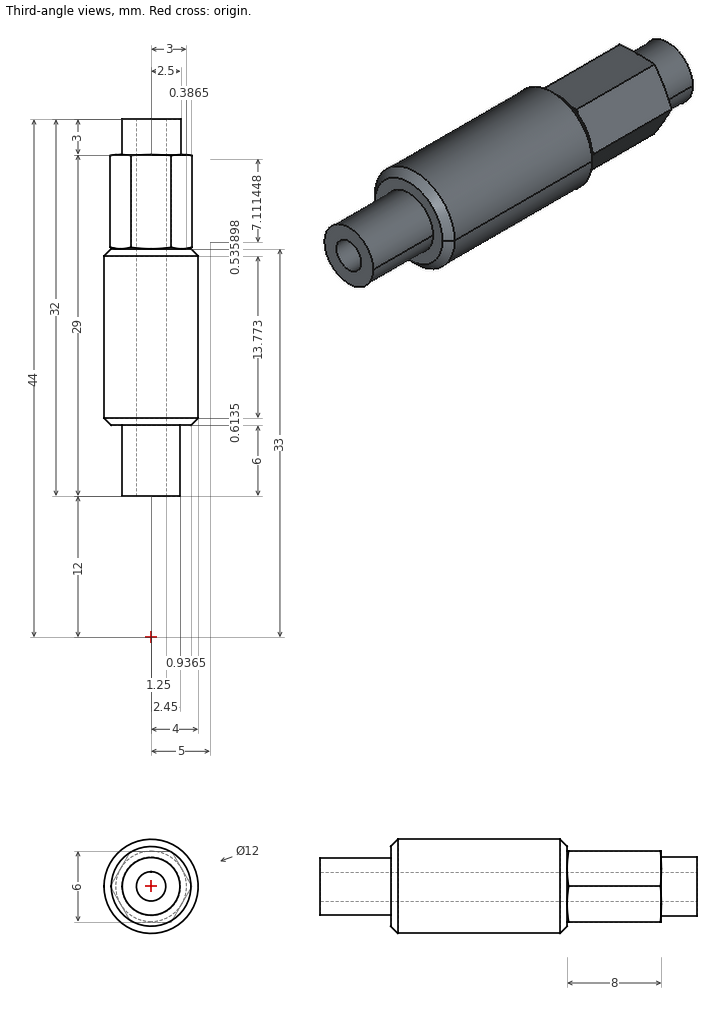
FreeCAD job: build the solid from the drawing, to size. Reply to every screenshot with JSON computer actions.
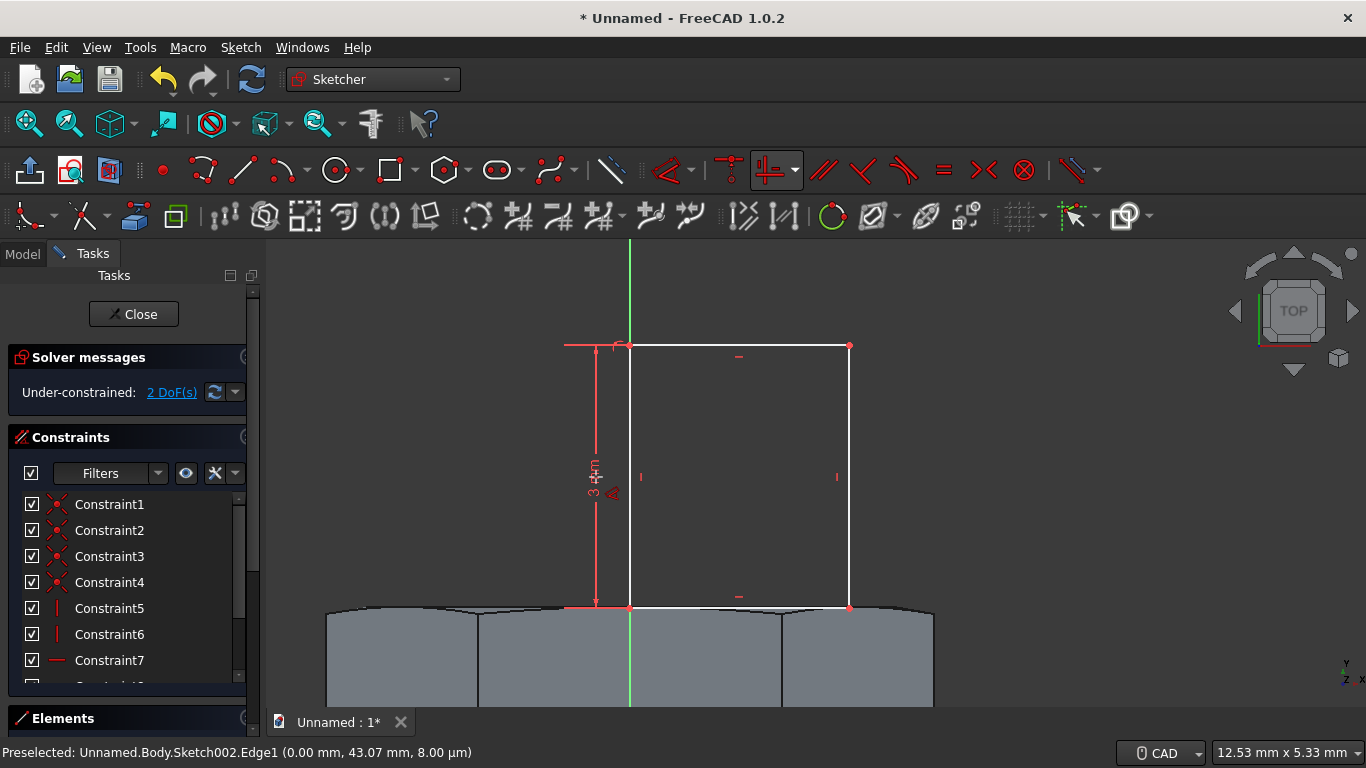
{"action": "left_click", "coordinate": [696, 608]}
{"action": "left_click", "coordinate": [739, 642]}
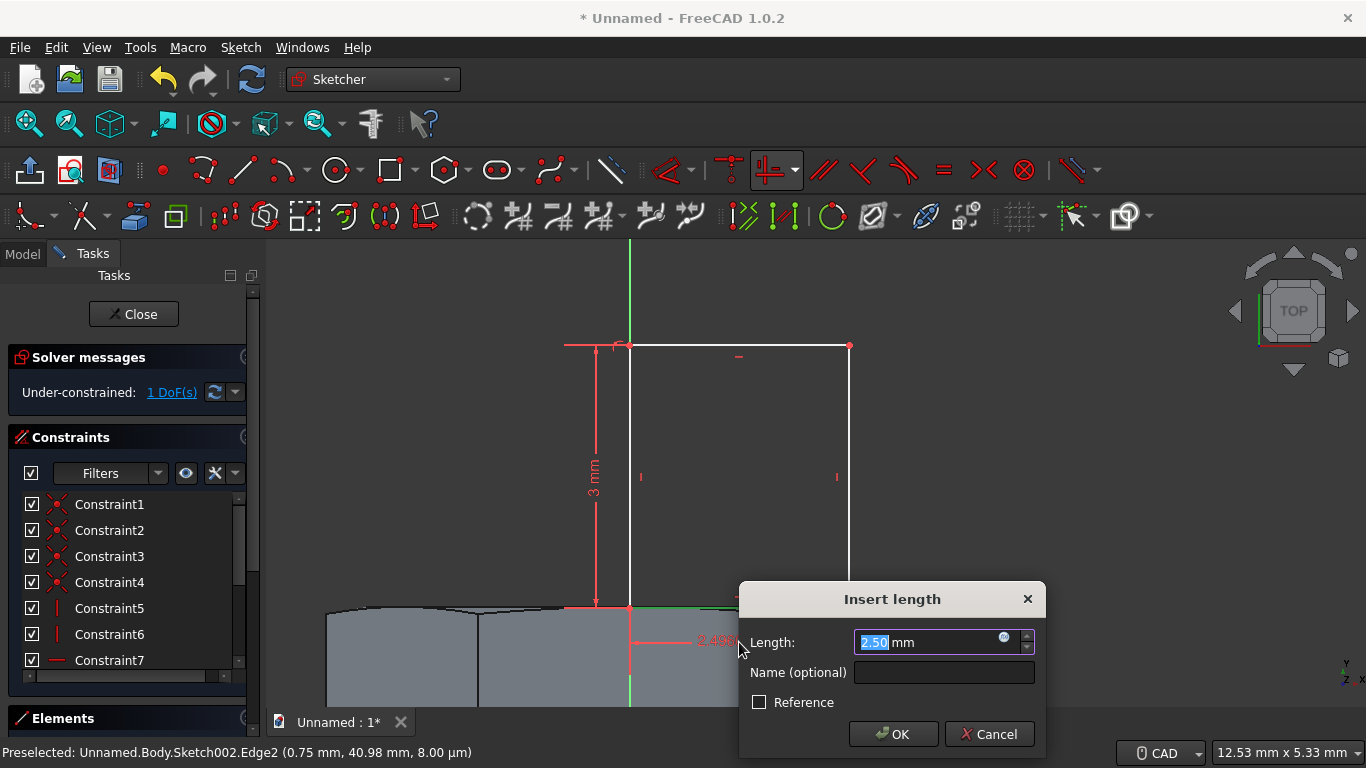
{"action": "type", "text": "2.5"}
{"action": "key", "text": "Return"}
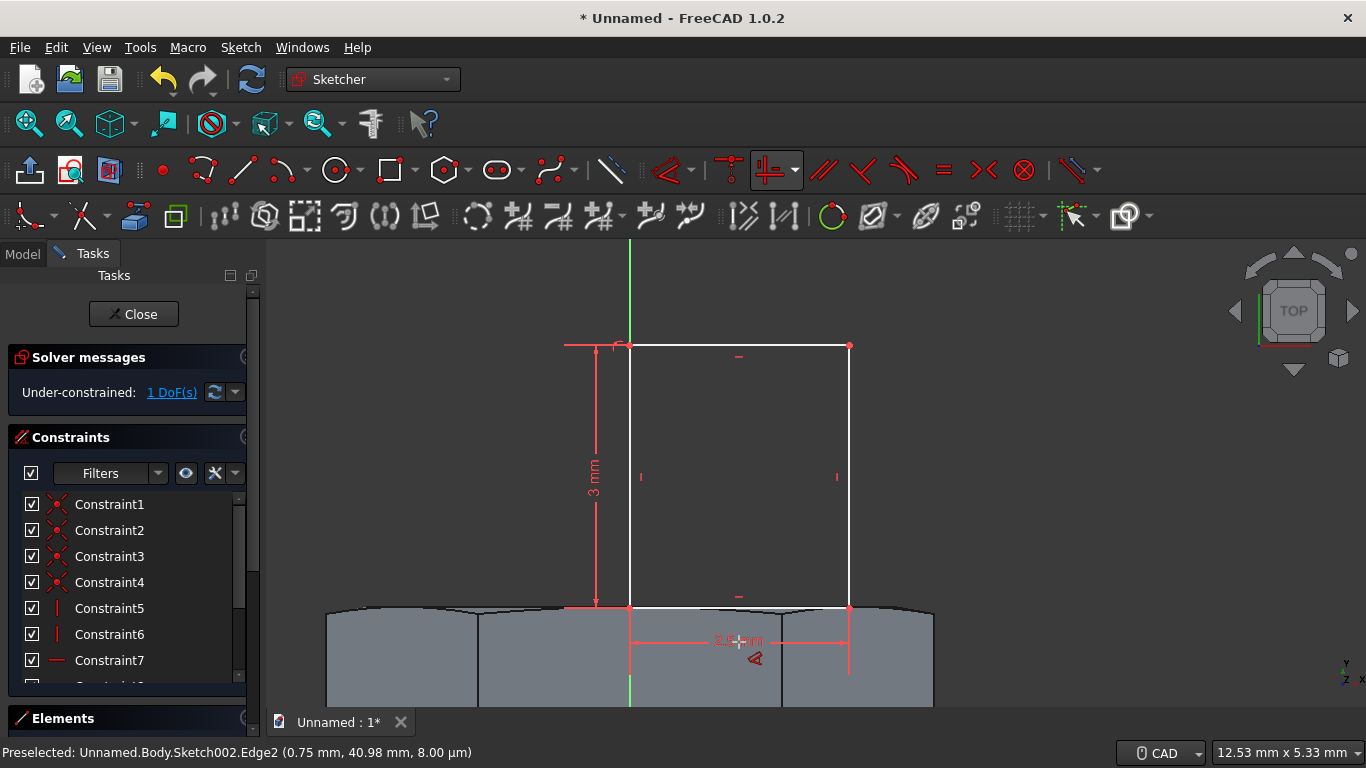
{"action": "left_click", "coordinate": [630, 345]}
{"action": "left_click", "coordinate": [596, 512]}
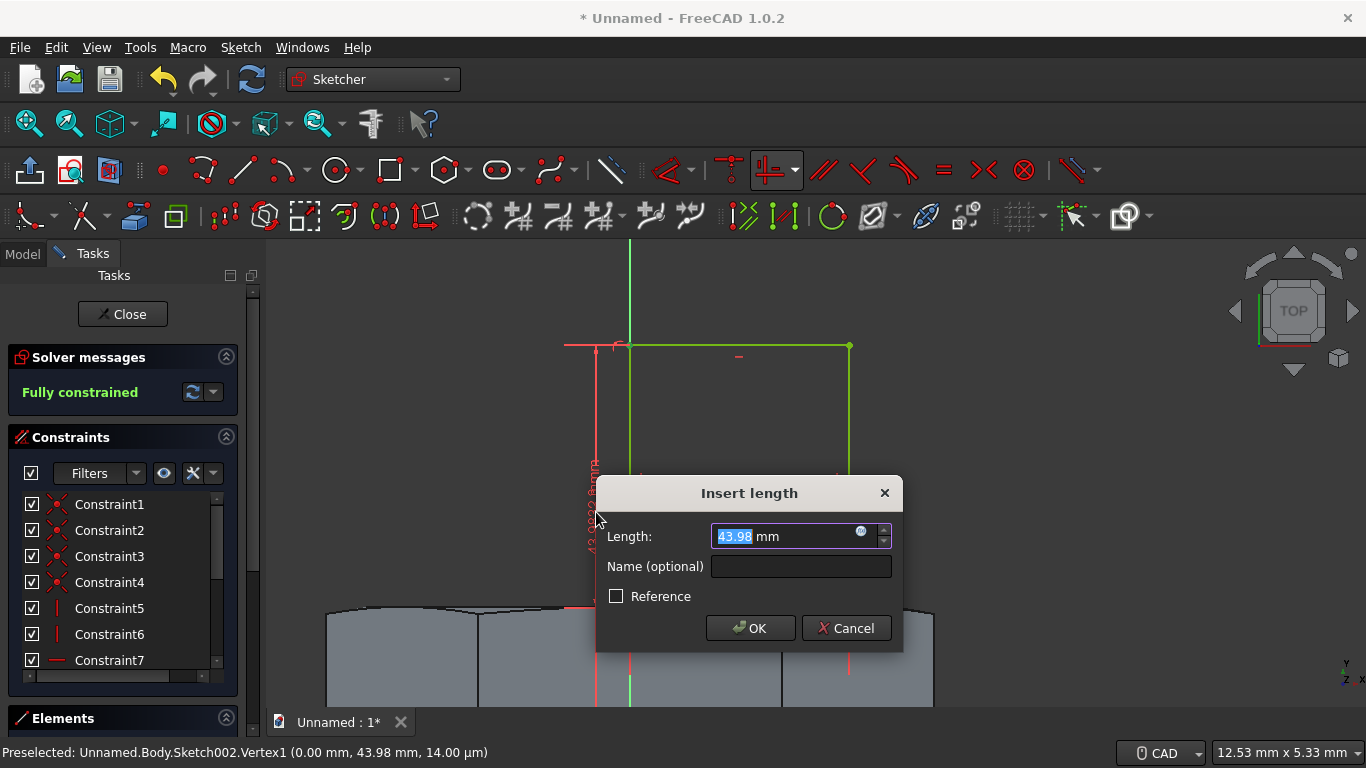
{"action": "type", "text": "44"}
{"action": "key", "text": "Return"}
{"action": "key", "text": "Escape"}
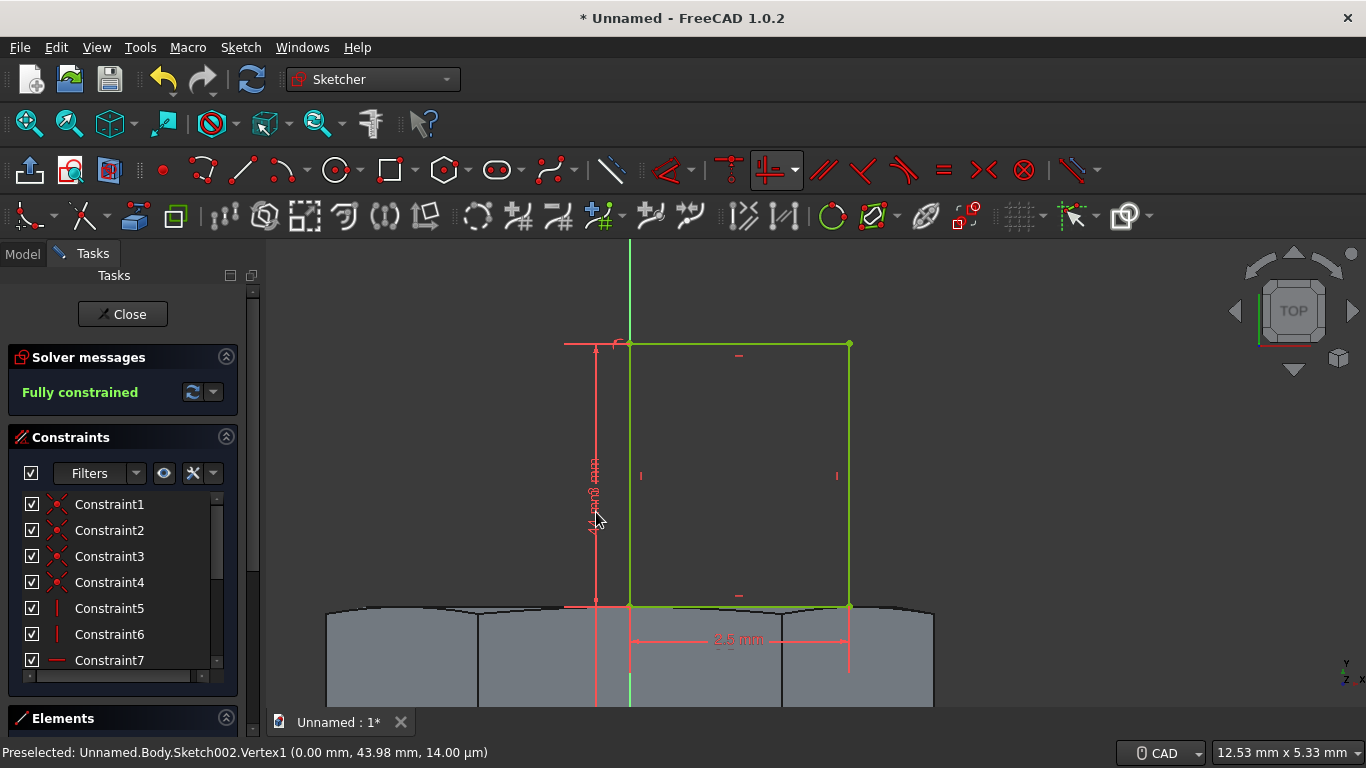
{"action": "left_click", "coordinate": [123, 314]}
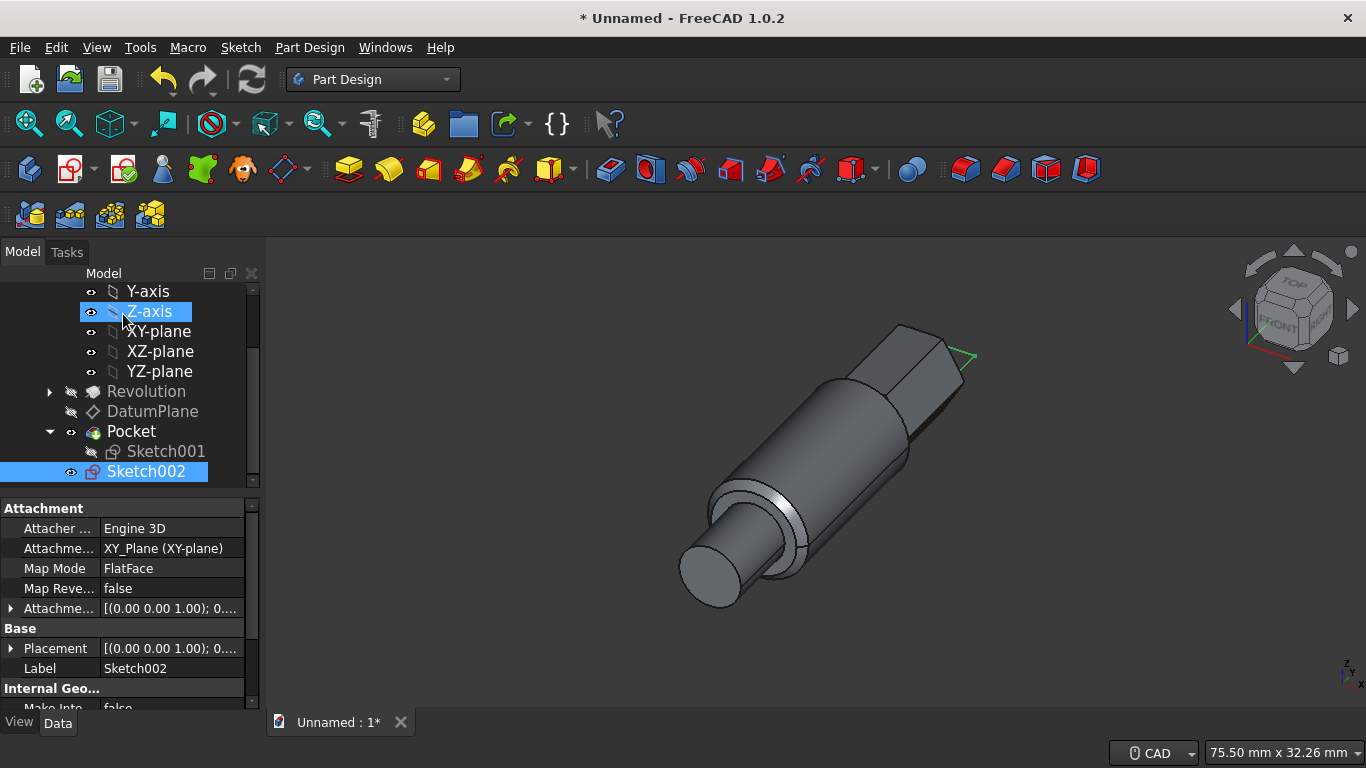
{"action": "left_click", "coordinate": [390, 170]}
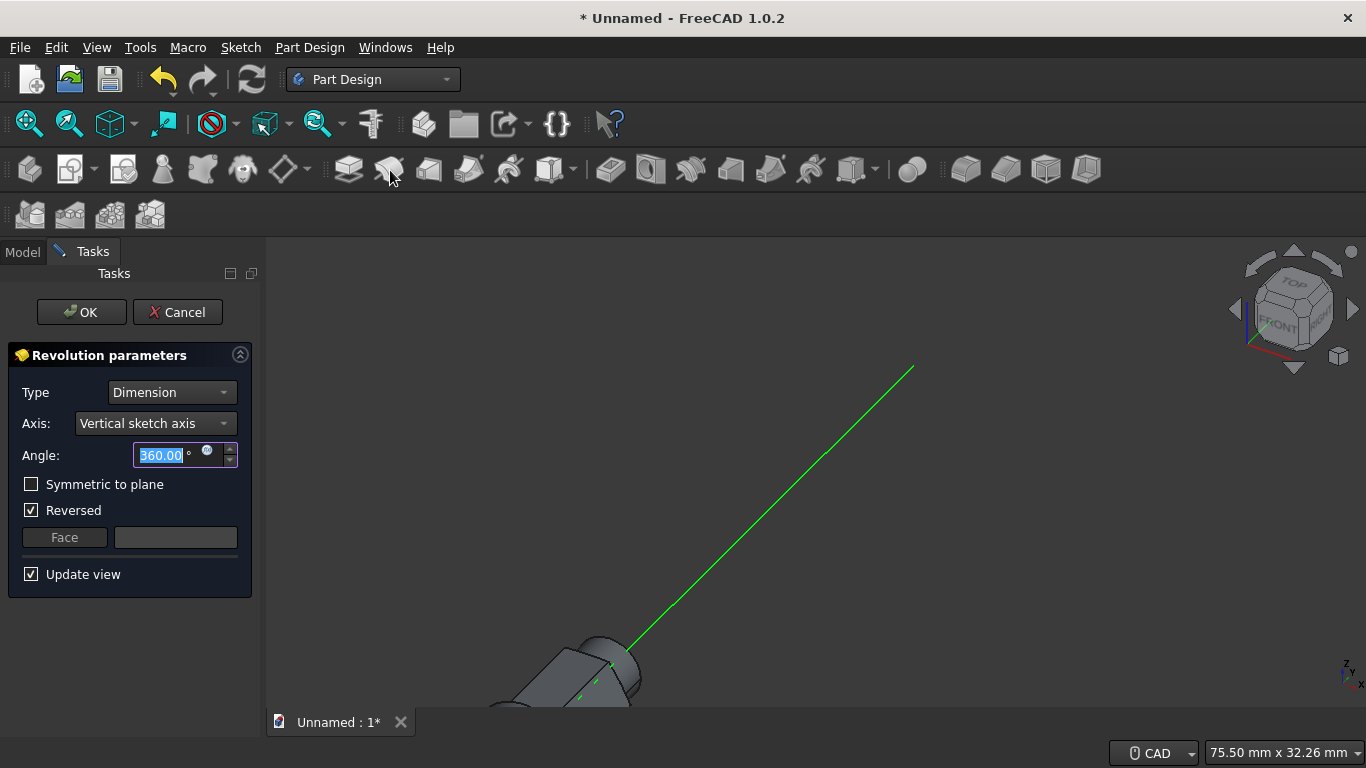
{"action": "left_click", "coordinate": [82, 312]}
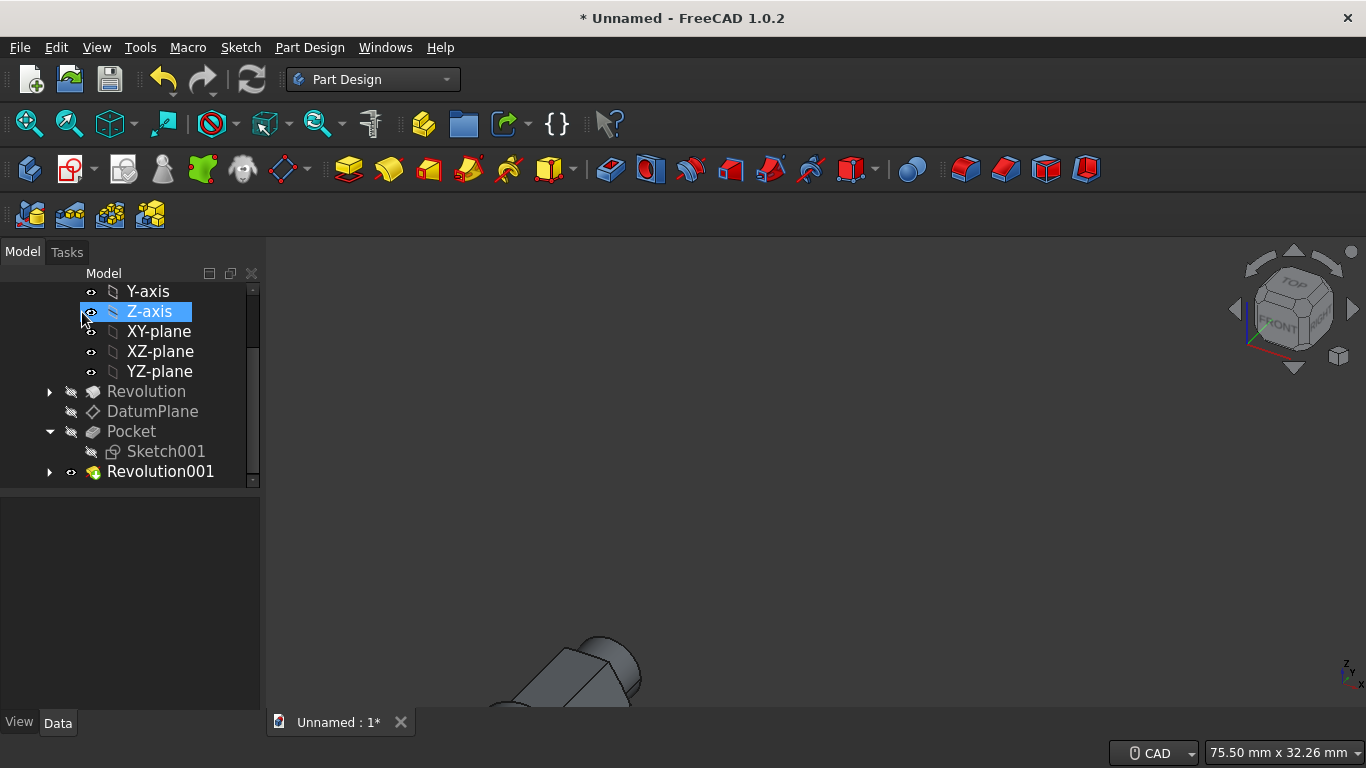
{"action": "left_click", "coordinate": [30, 124]}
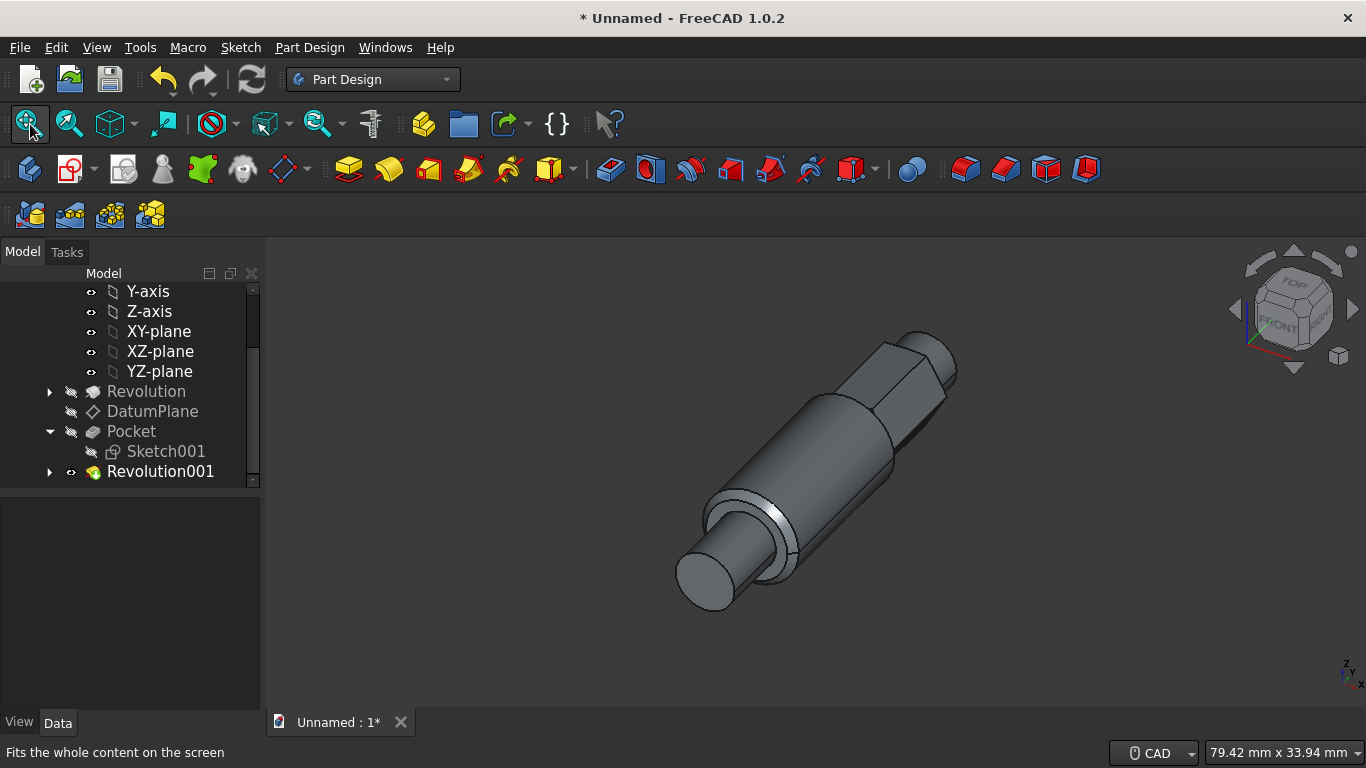
{"action": "left_click", "coordinate": [70, 170]}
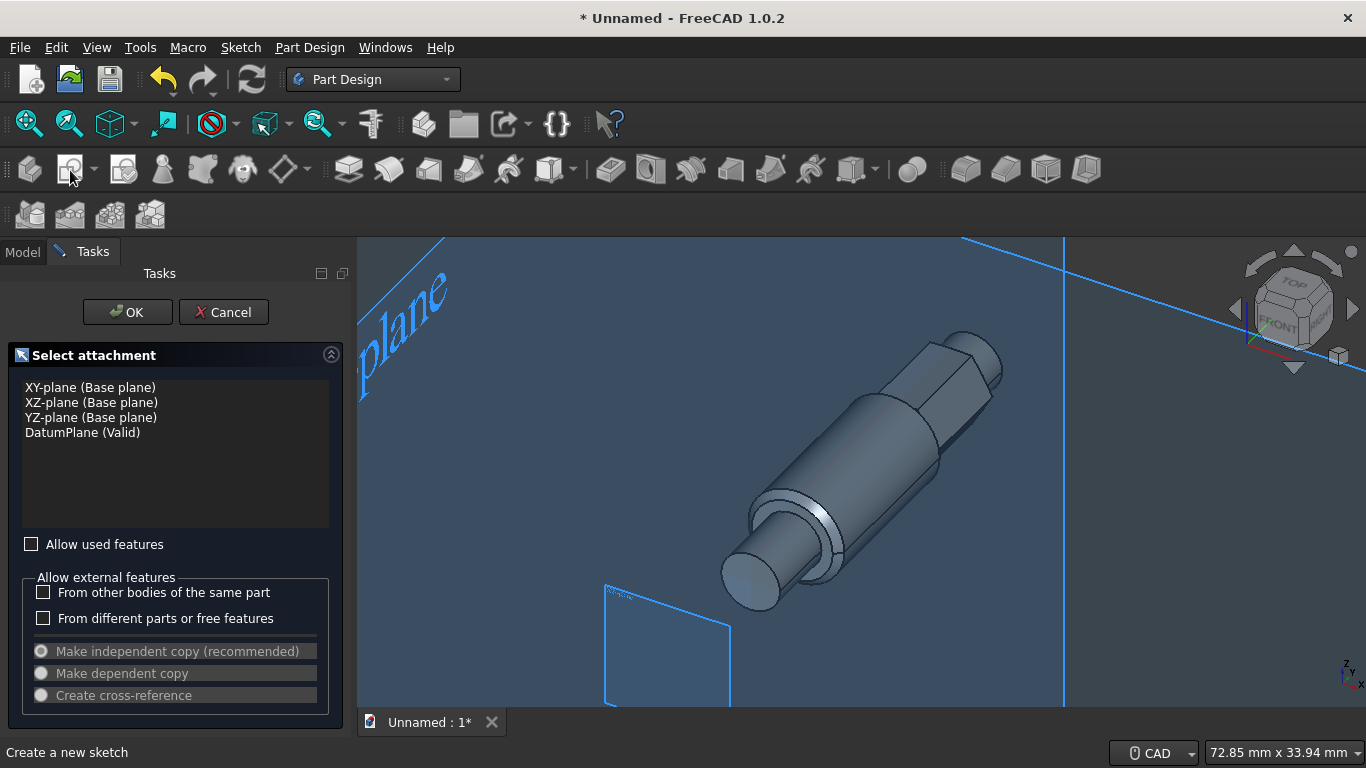
{"action": "left_click", "coordinate": [82, 388]}